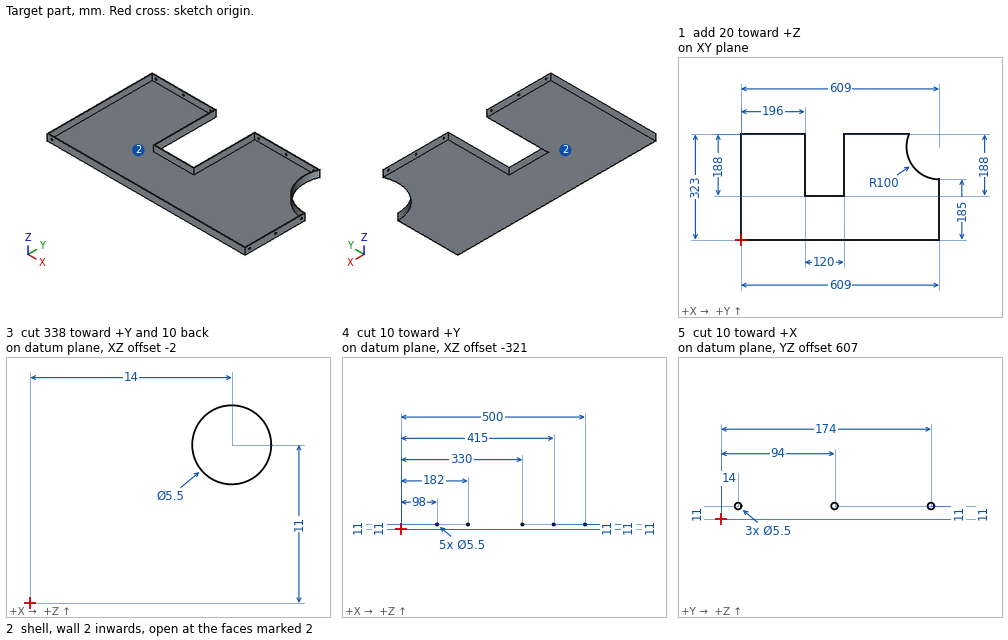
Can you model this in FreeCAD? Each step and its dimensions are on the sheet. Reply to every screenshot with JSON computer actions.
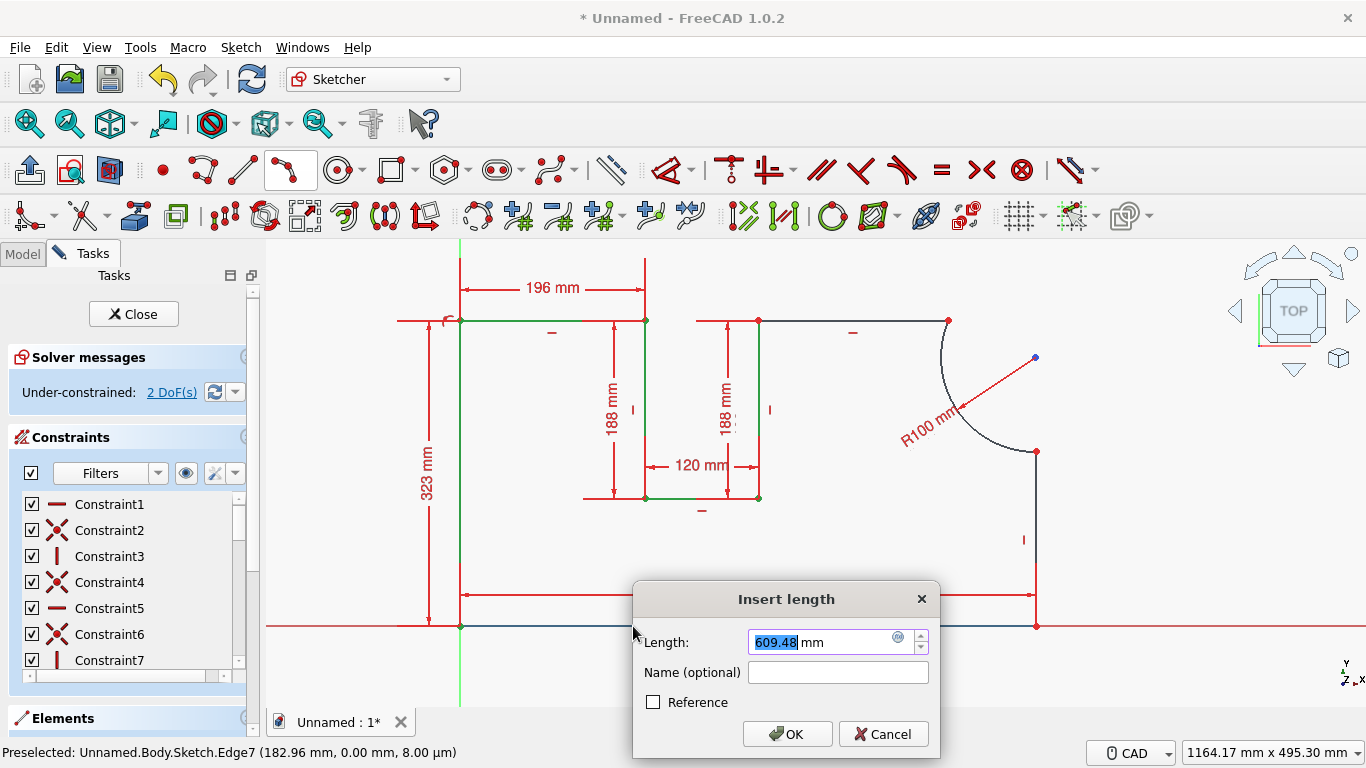
{"action": "type", "text": "609"}
{"action": "key", "text": "Return"}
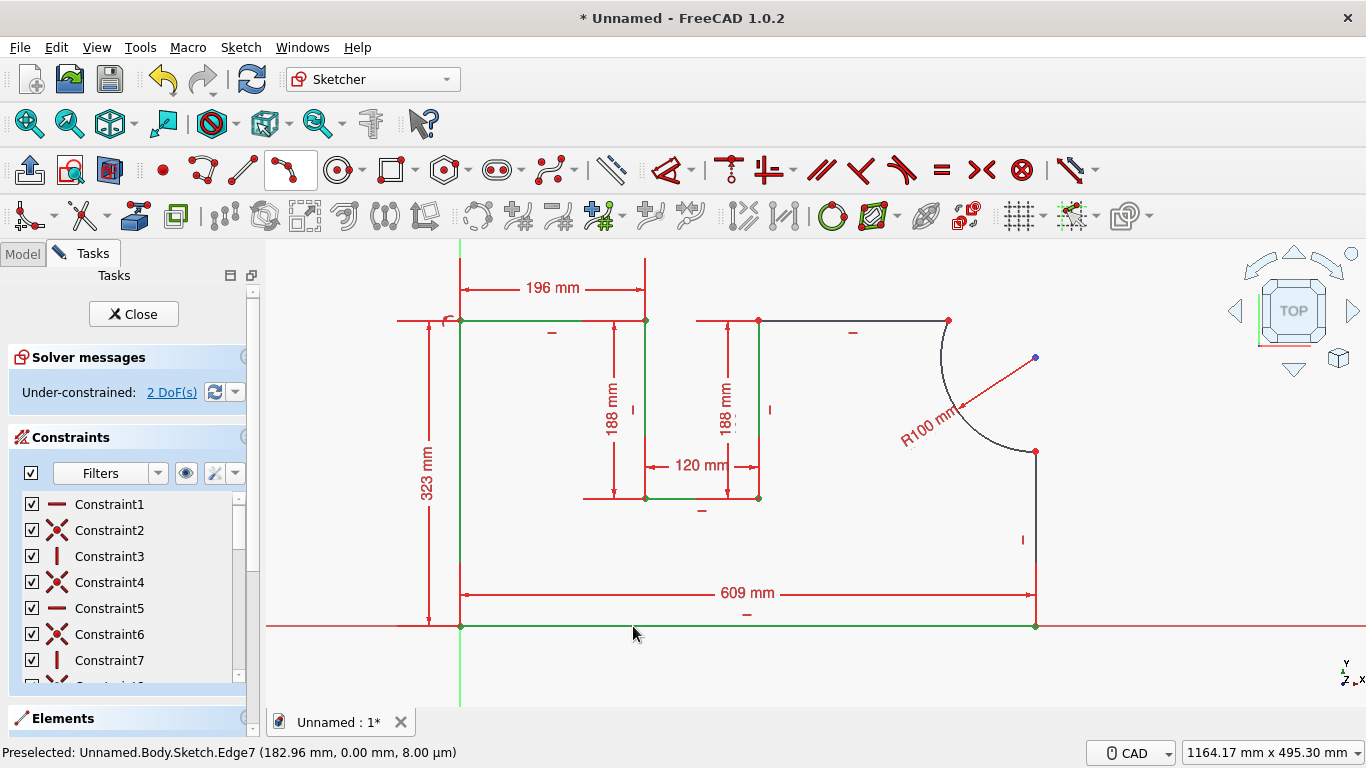
{"action": "left_click", "coordinate": [1036, 574]}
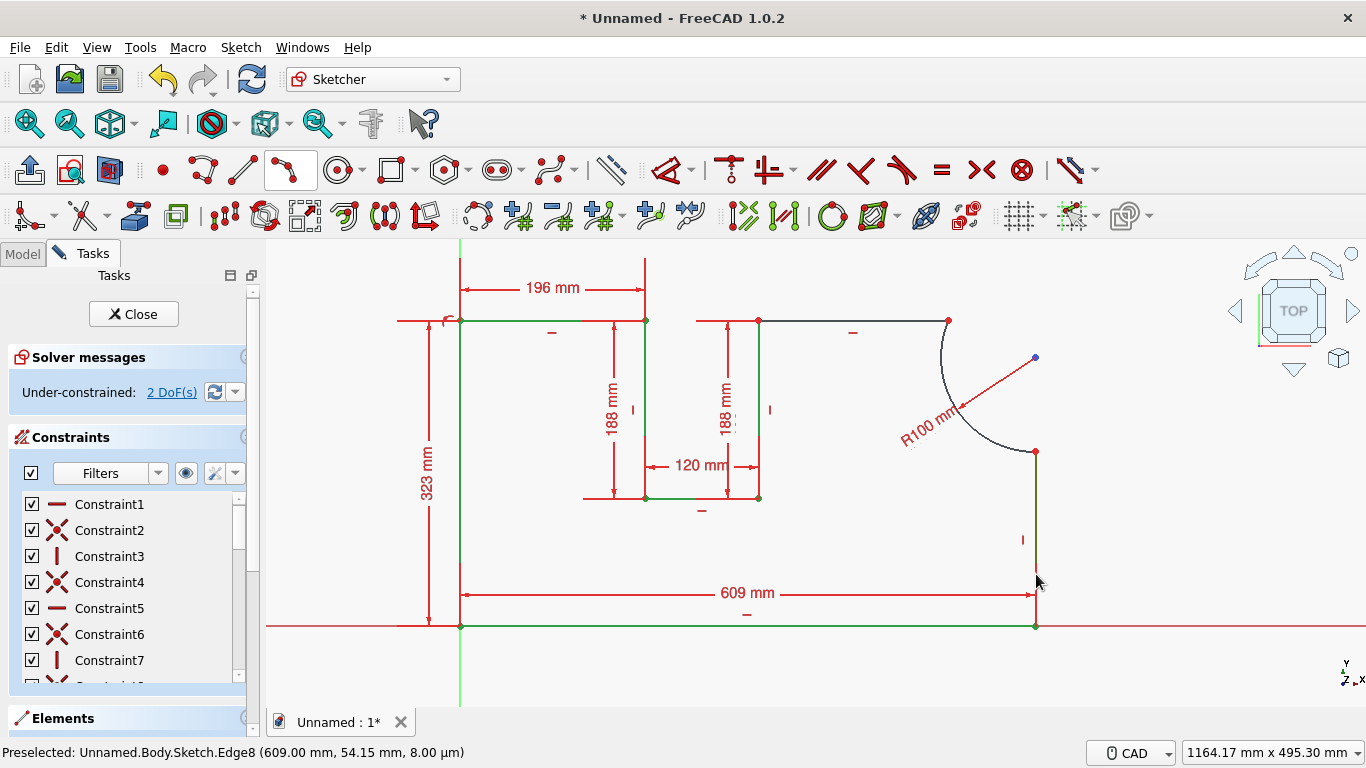
{"action": "key", "text": "i"}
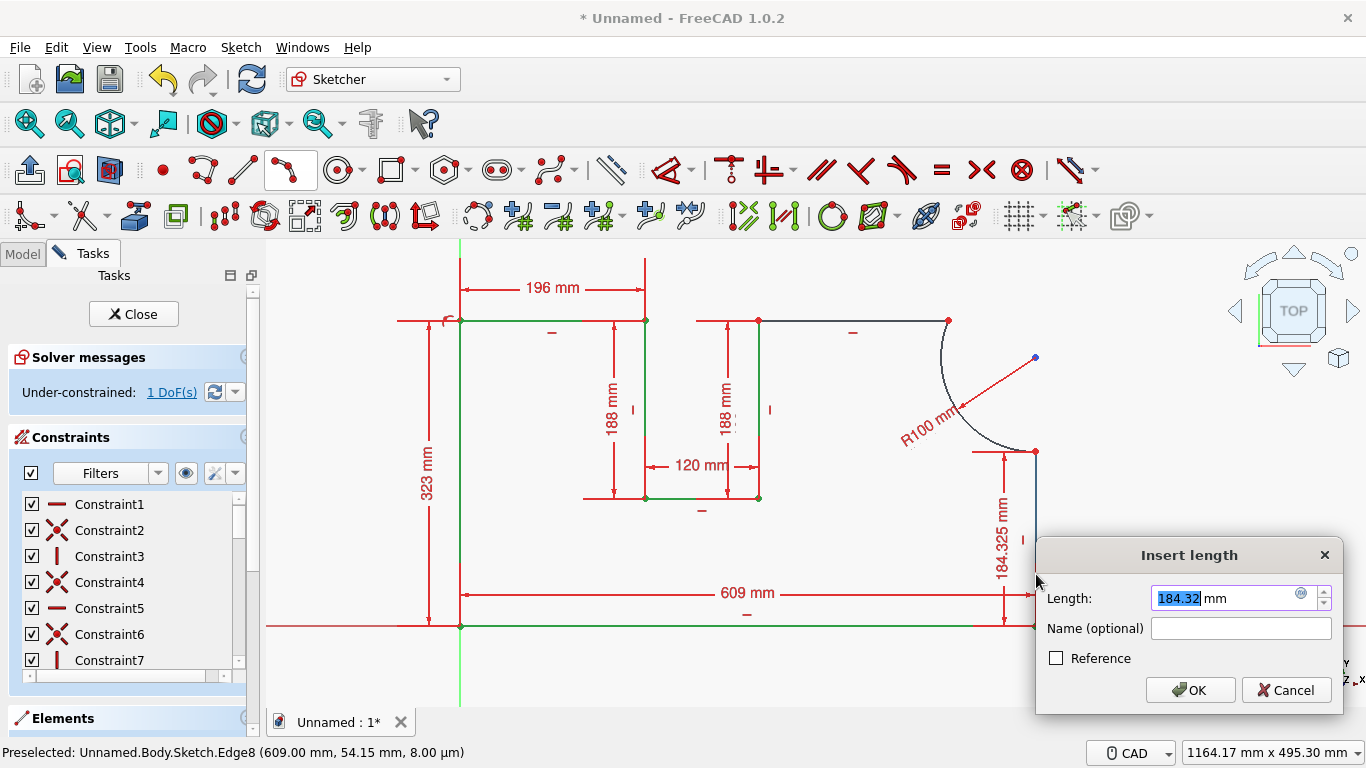
{"action": "type", "text": "185"}
{"action": "key", "text": "Return"}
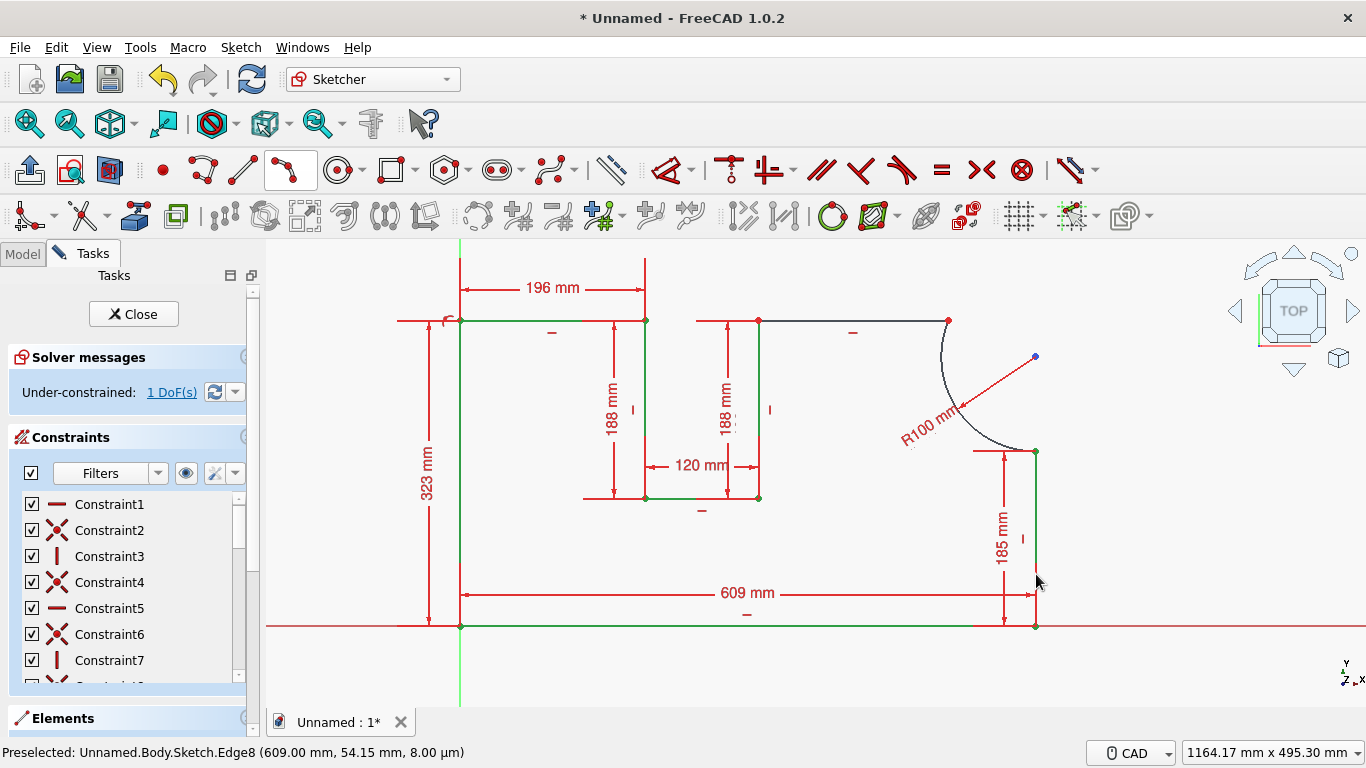
{"action": "left_click", "coordinate": [1036, 357]}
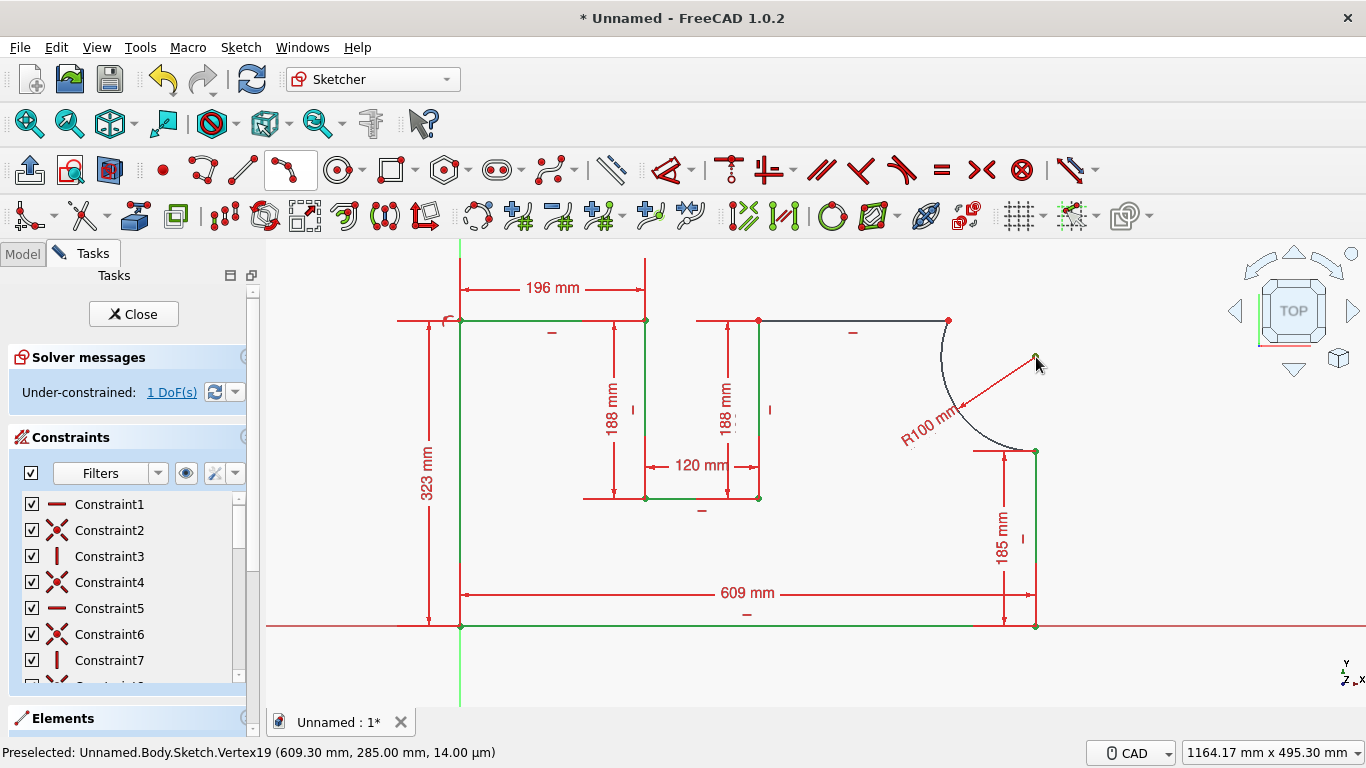
{"action": "key", "text": "l"}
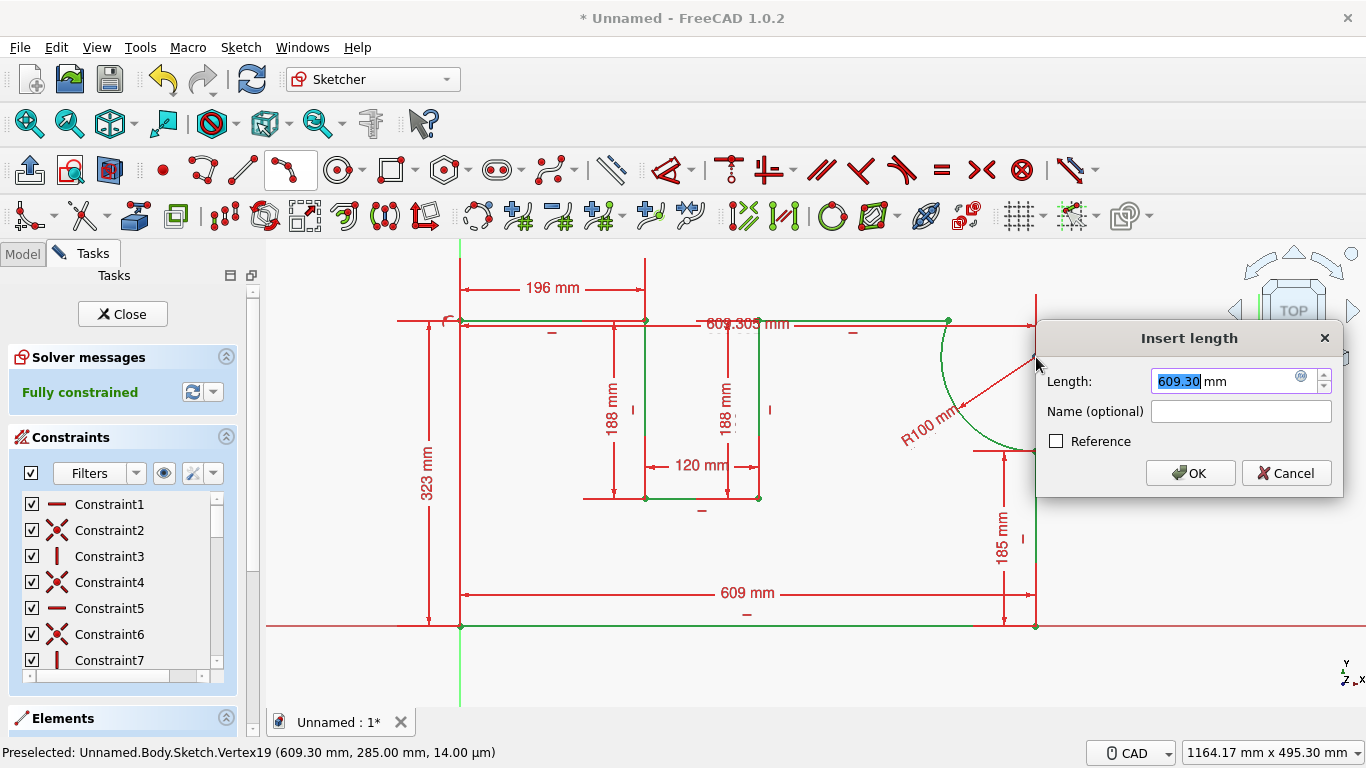
{"action": "type", "text": "609"}
{"action": "key", "text": "Return"}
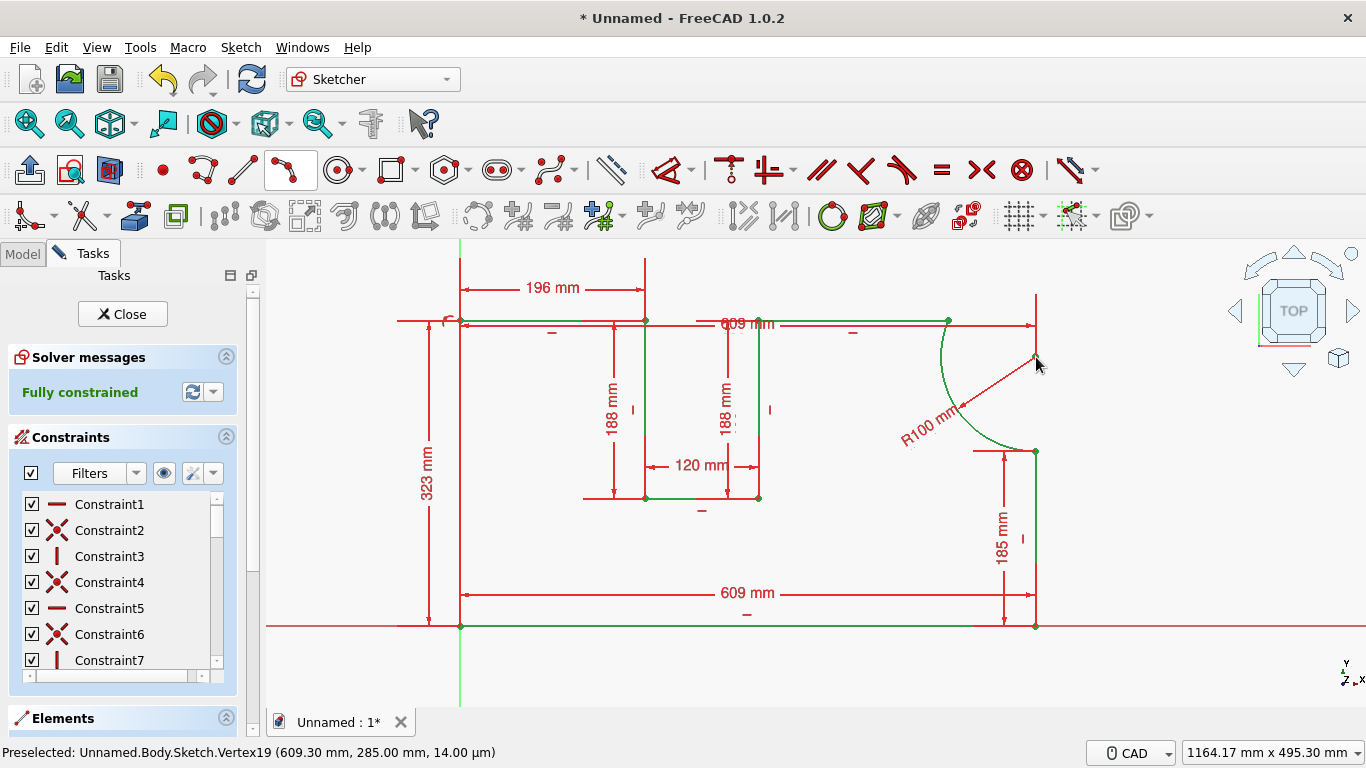
{"action": "left_click", "coordinate": [123, 314]}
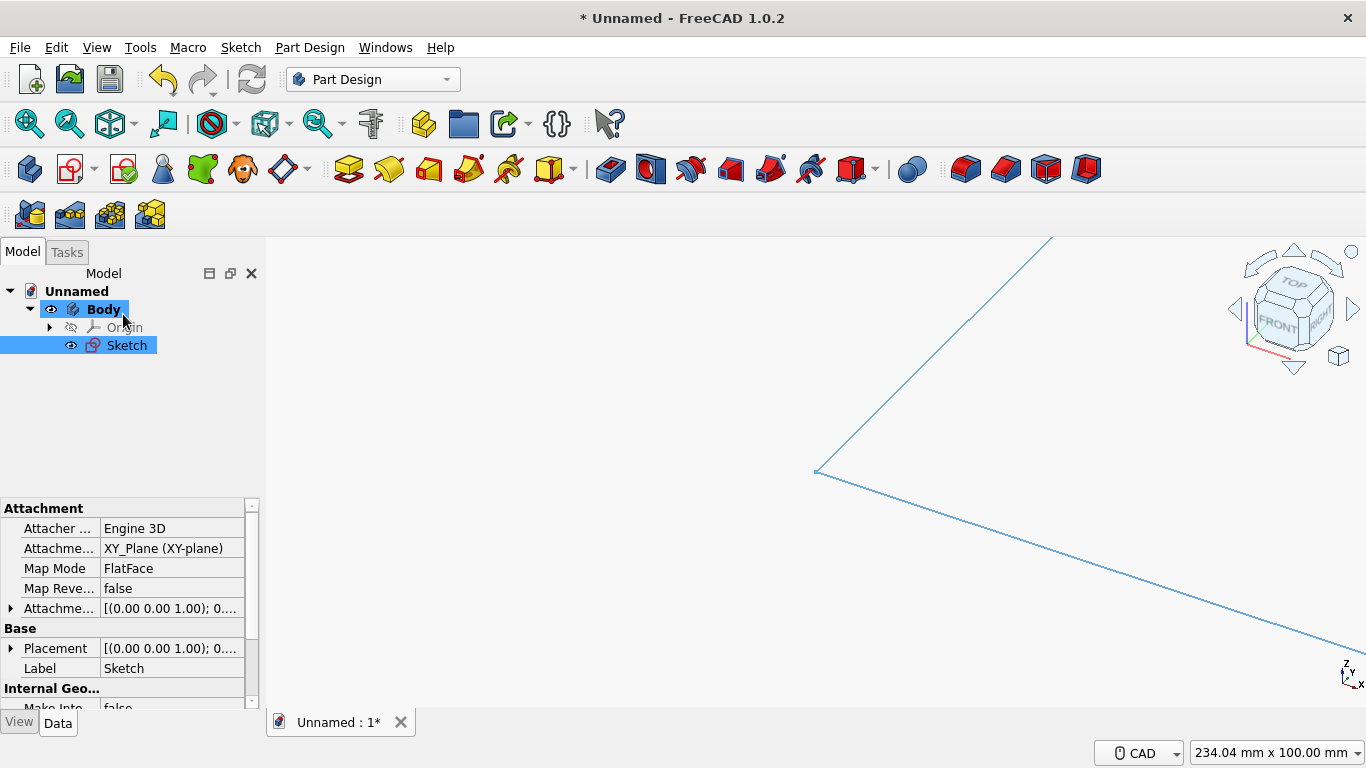
{"action": "left_click", "coordinate": [350, 170]}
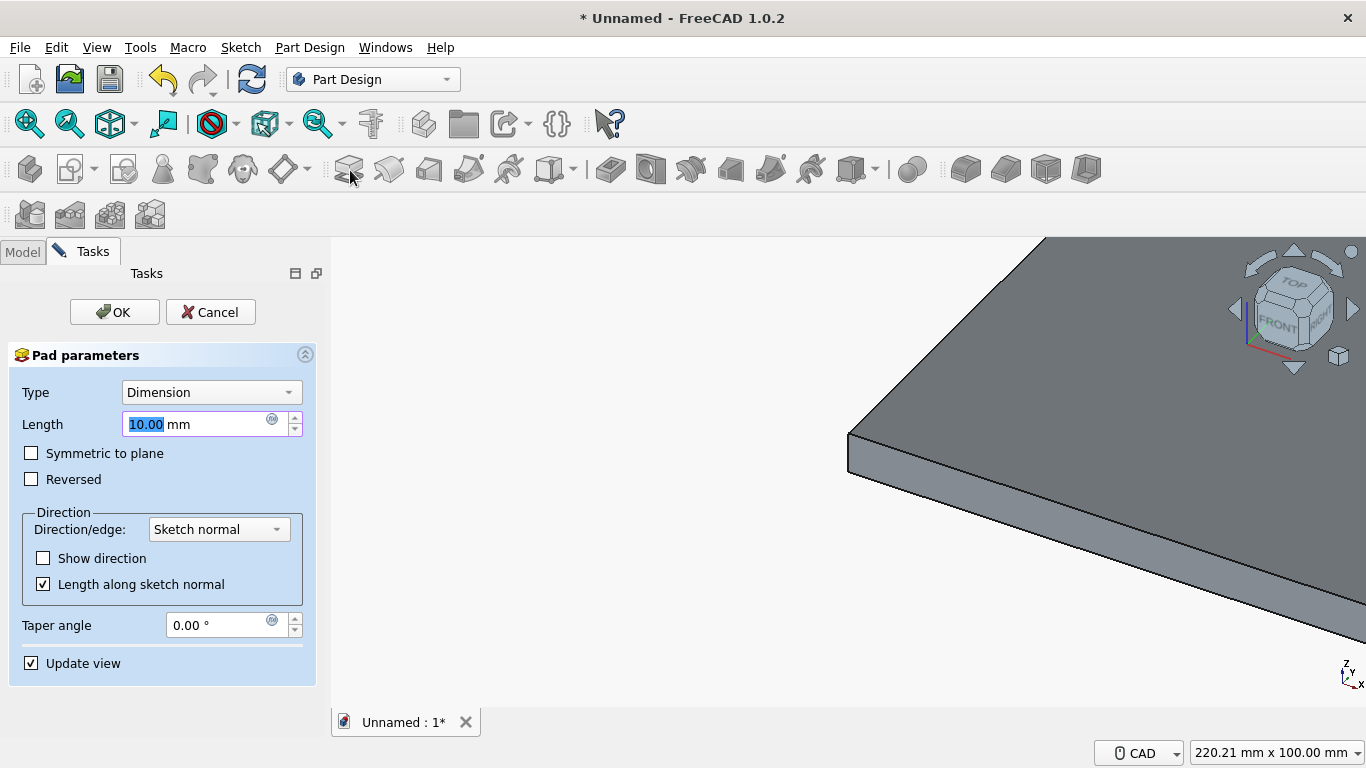
{"action": "type", "text": "20"}
{"action": "key", "text": "Tab"}